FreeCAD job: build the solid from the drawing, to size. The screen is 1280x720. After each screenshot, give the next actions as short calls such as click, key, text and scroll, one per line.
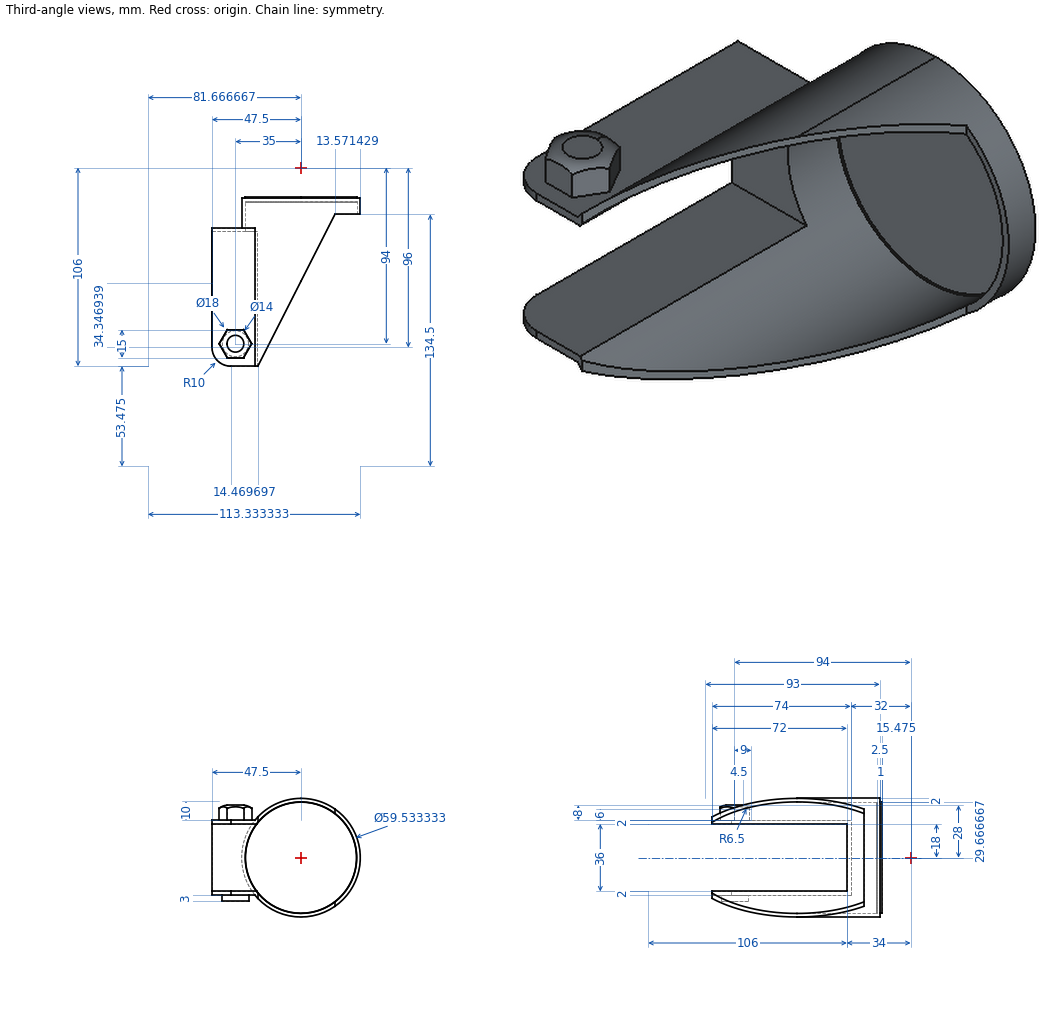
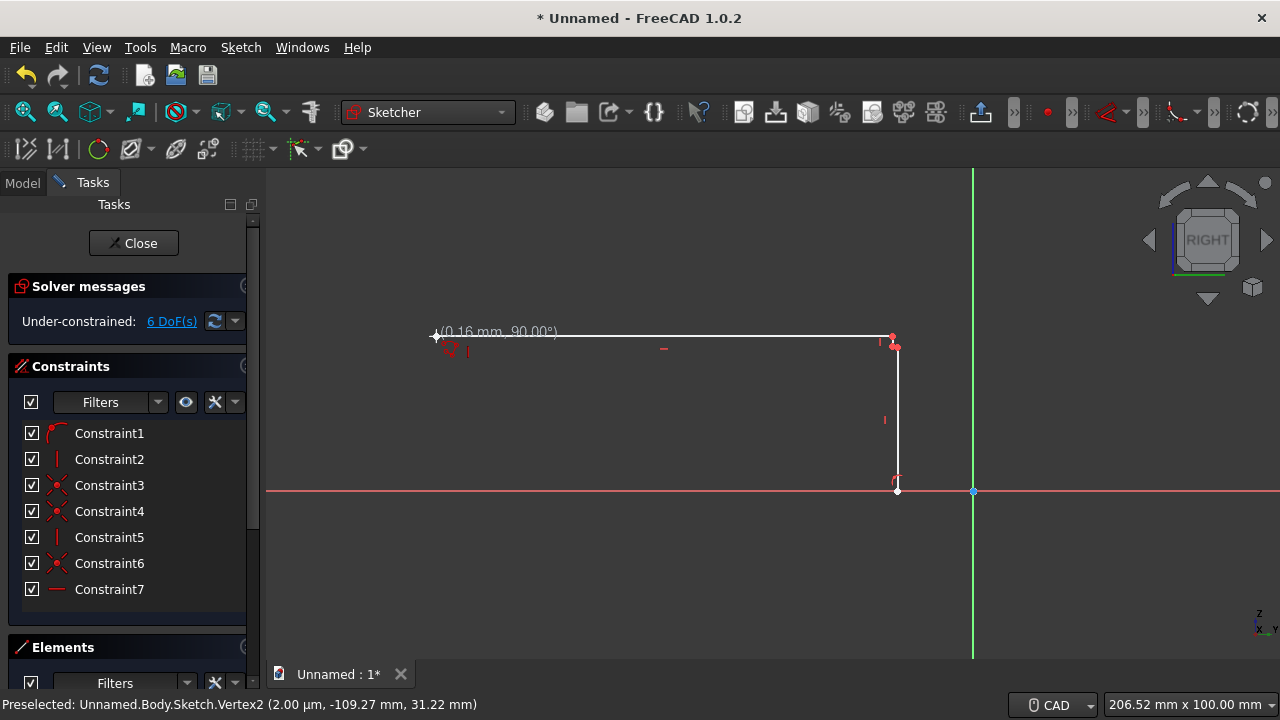
scroll(436, 346, up, 3)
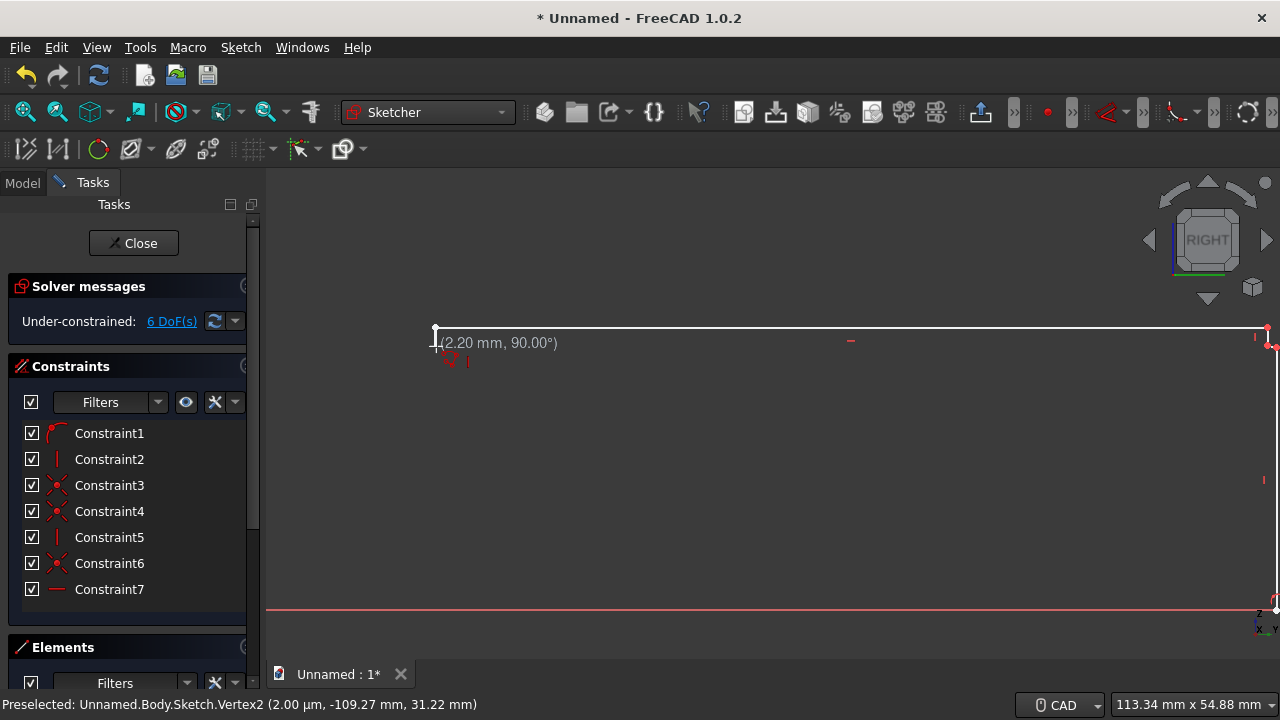
click(436, 345)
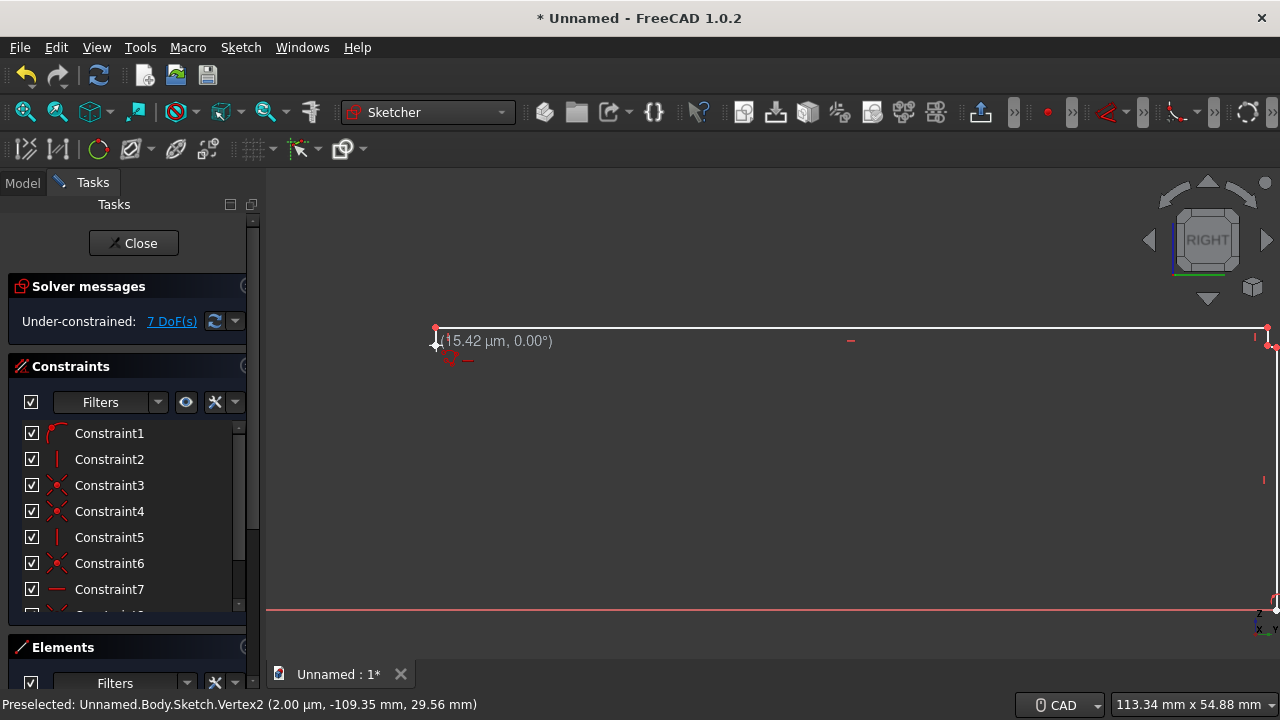
scroll(436, 346, down, 3)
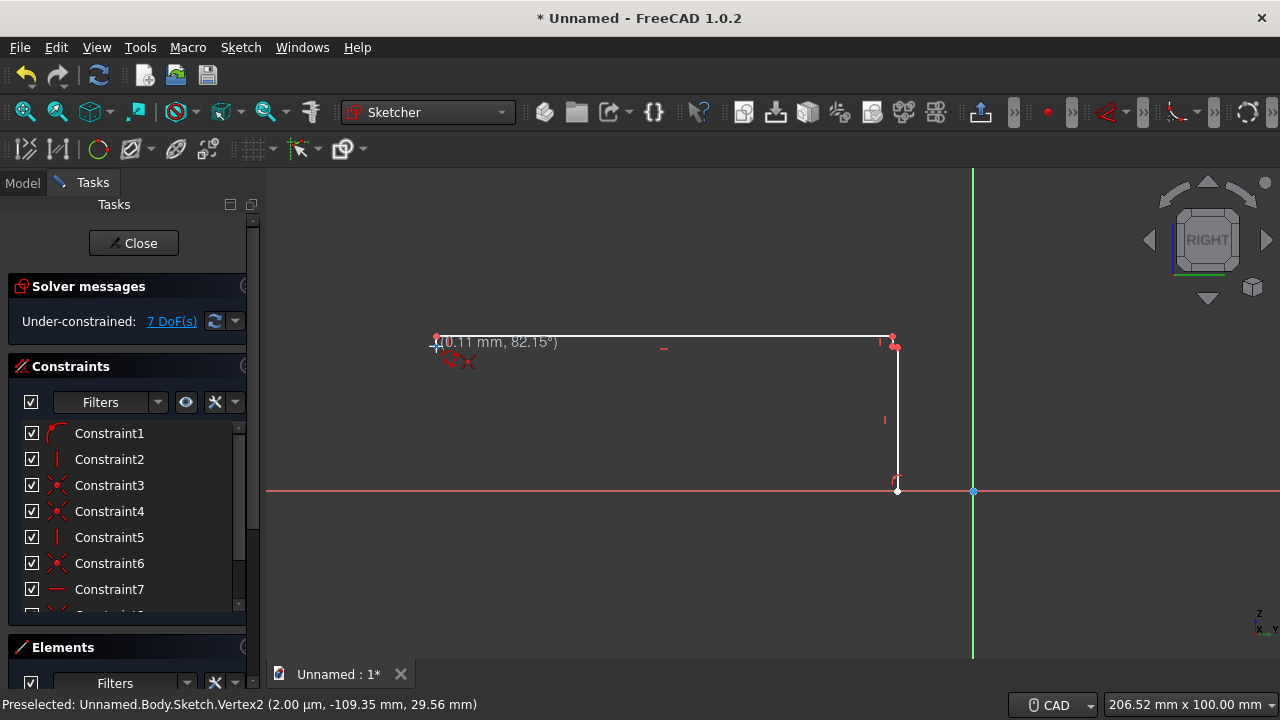
scroll(885, 346, up, 4)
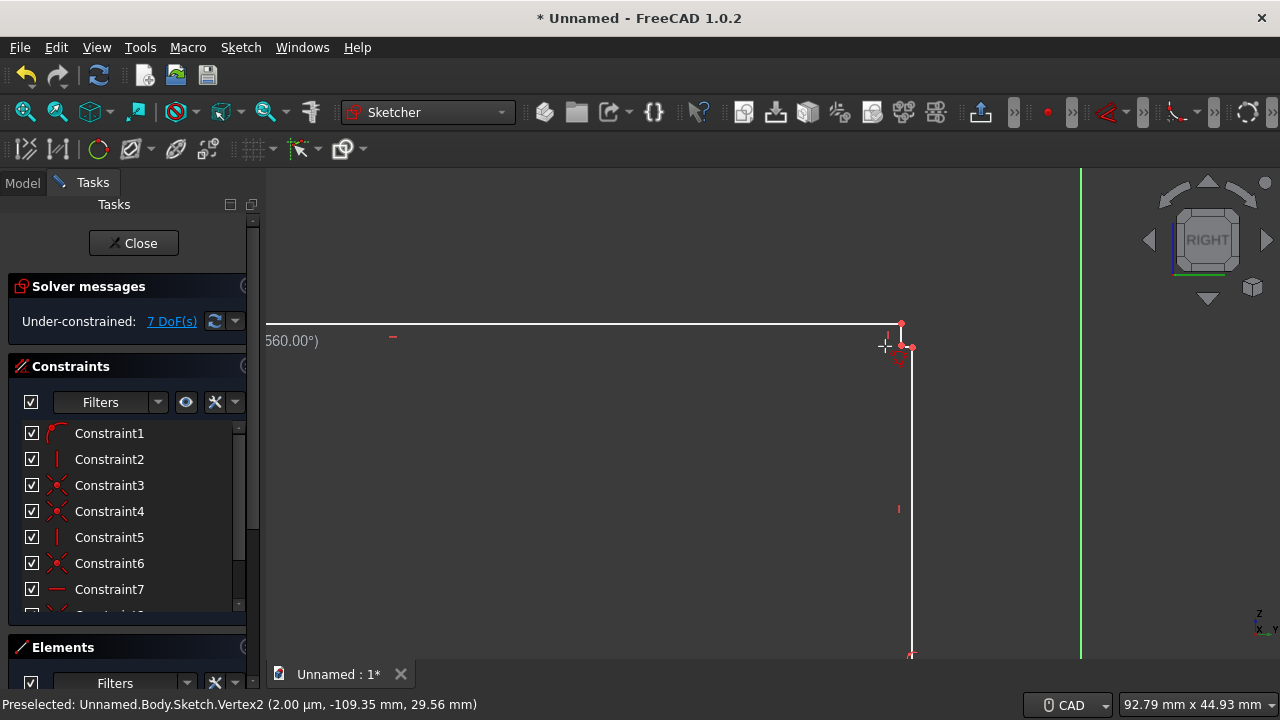
click(885, 345)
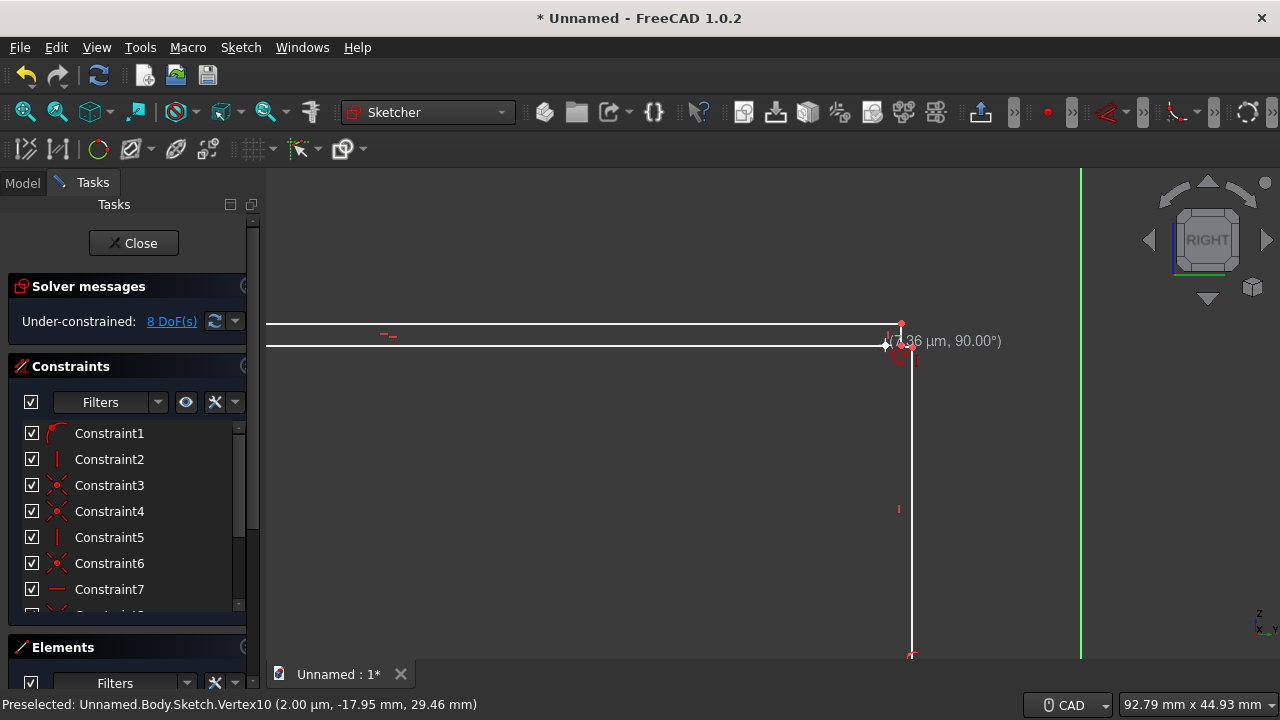
scroll(885, 346, down, 4)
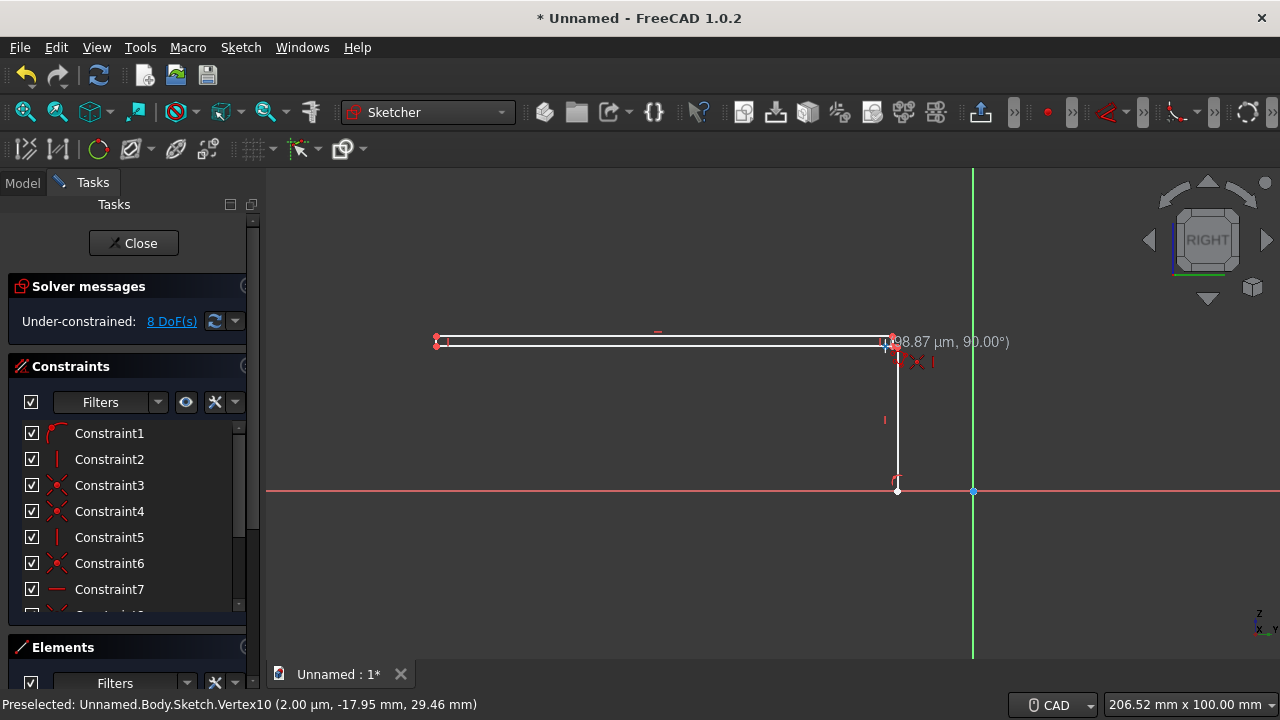
scroll(885, 491, up, 2)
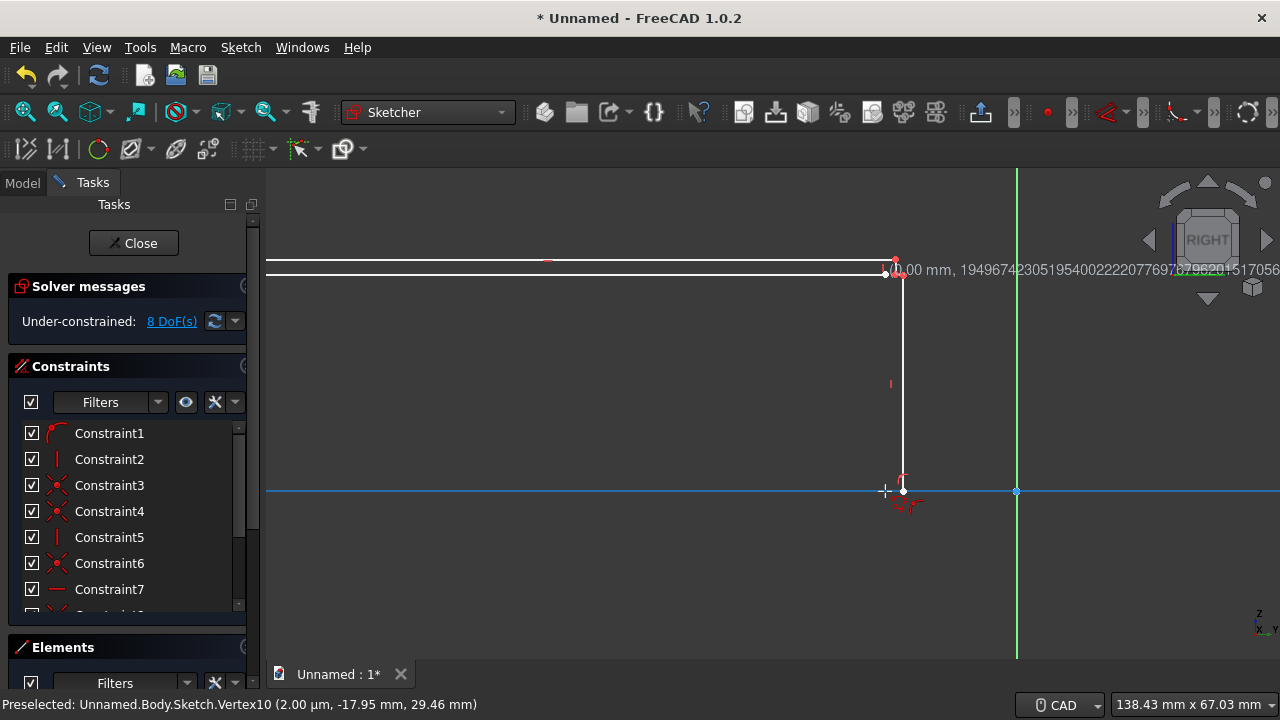
click(885, 482)
click(903, 491)
key(Escape)
key(Escape)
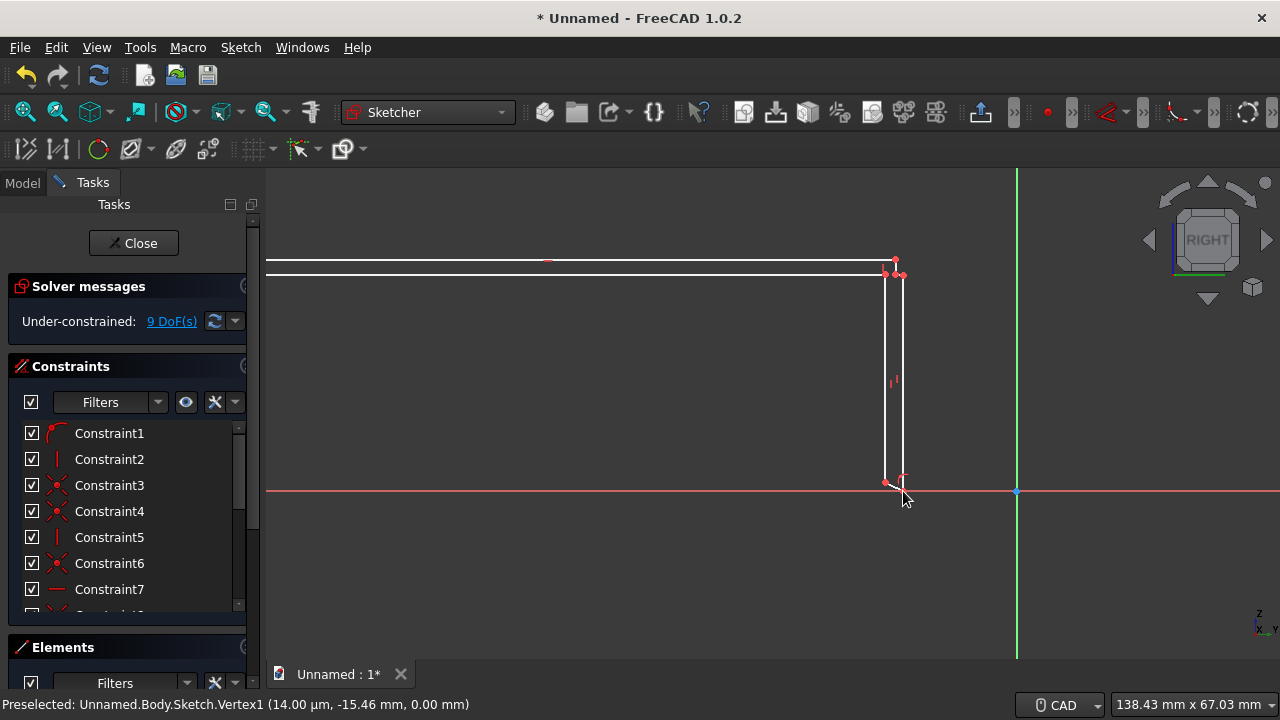
scroll(900, 275, up, 7)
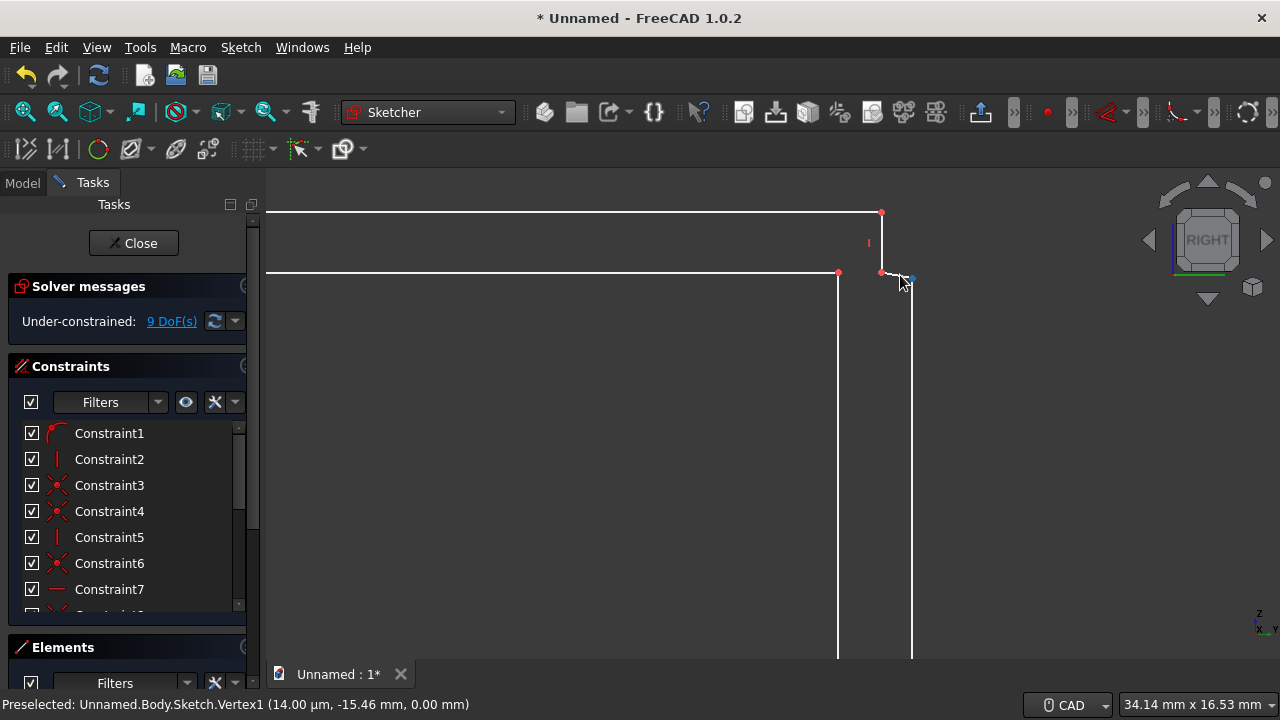
click(897, 275)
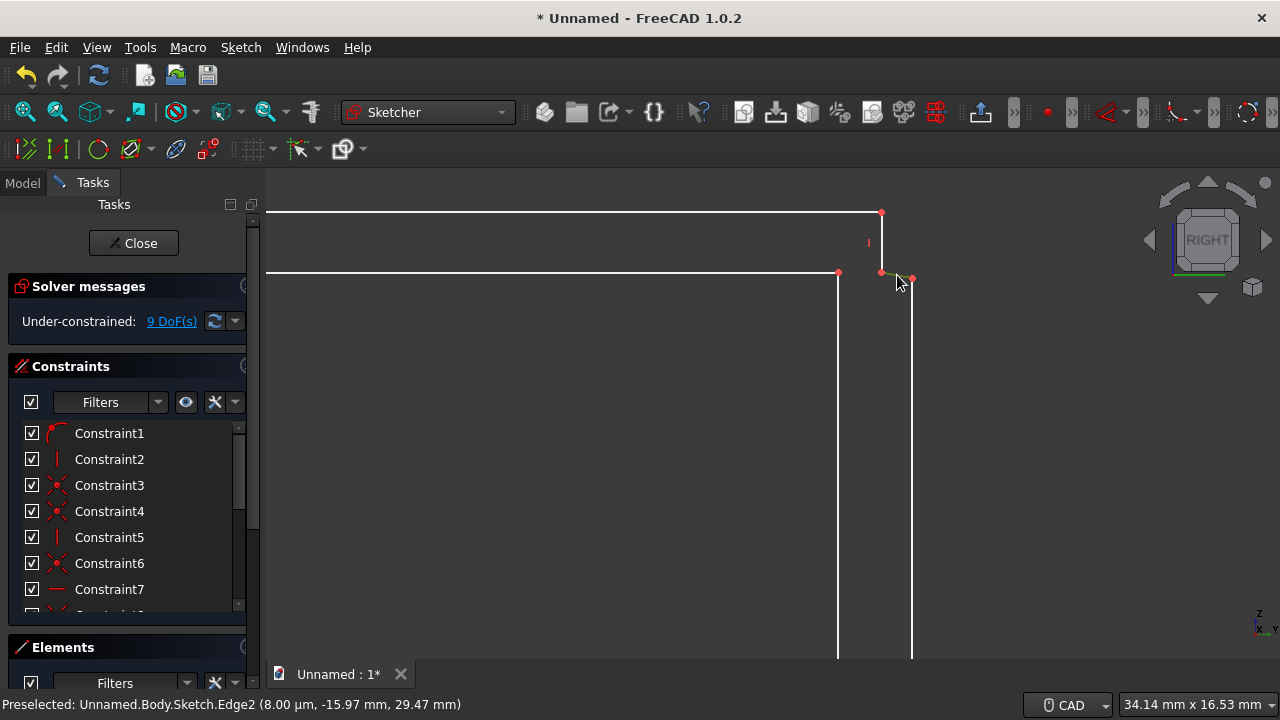
key(h)